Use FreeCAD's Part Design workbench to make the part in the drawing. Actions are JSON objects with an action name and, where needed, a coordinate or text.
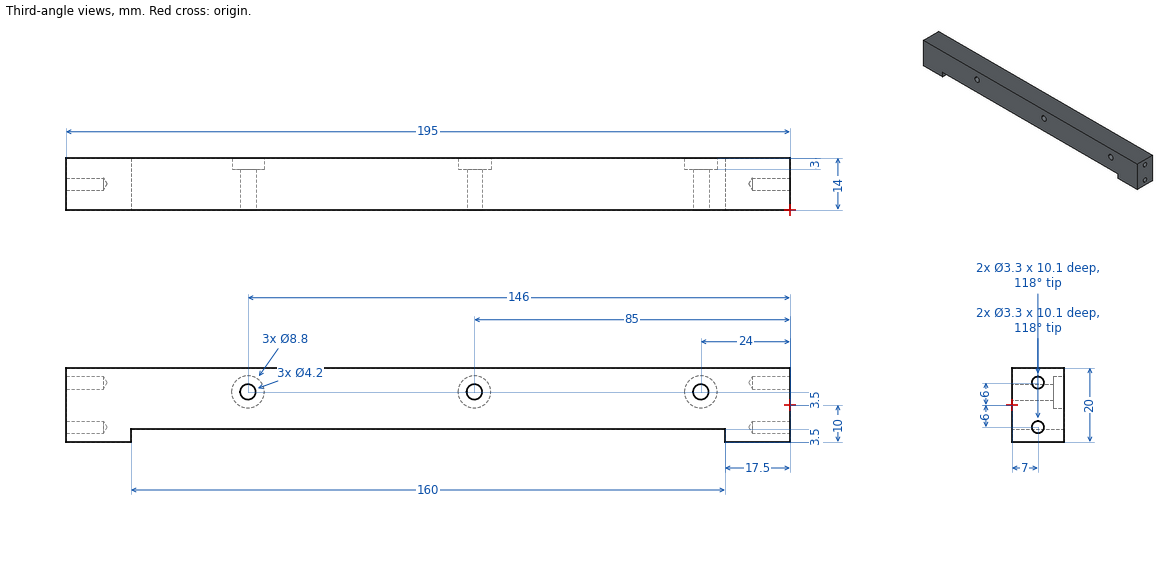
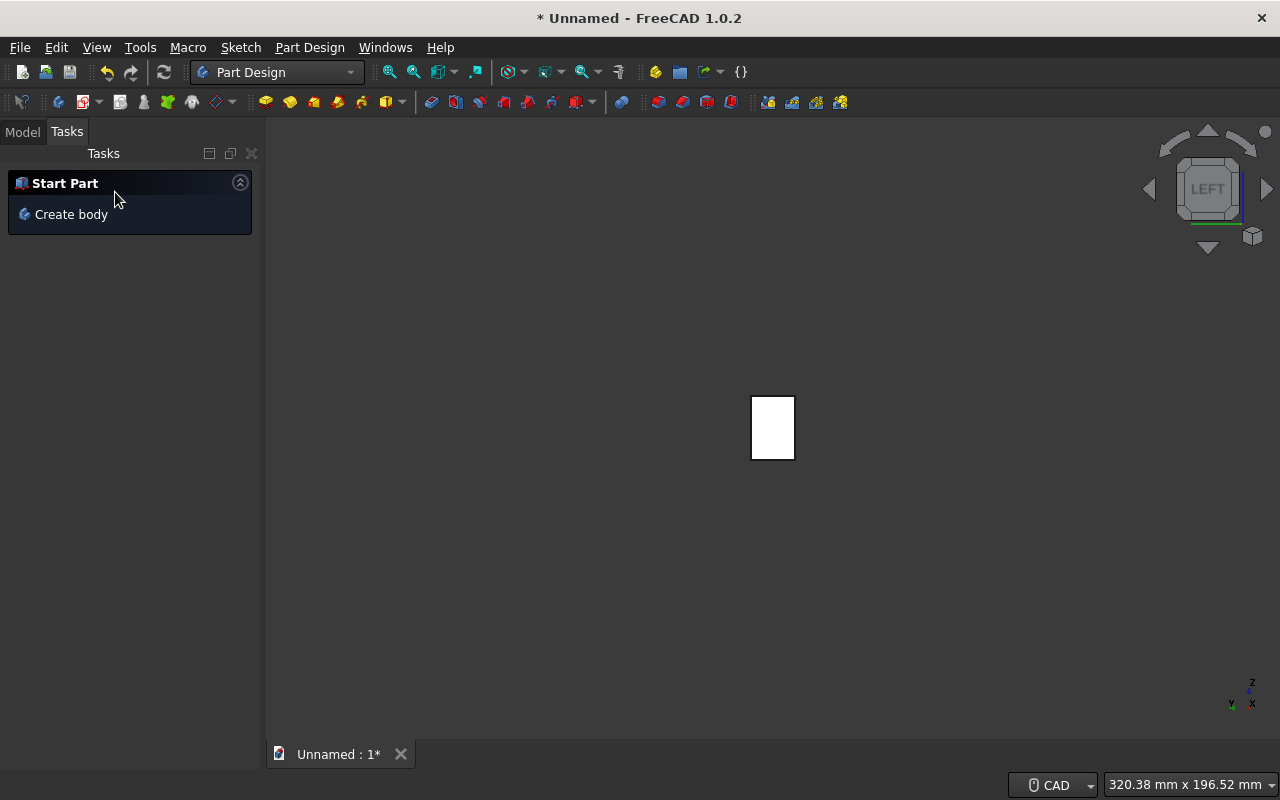
{"action": "key", "text": "v f"}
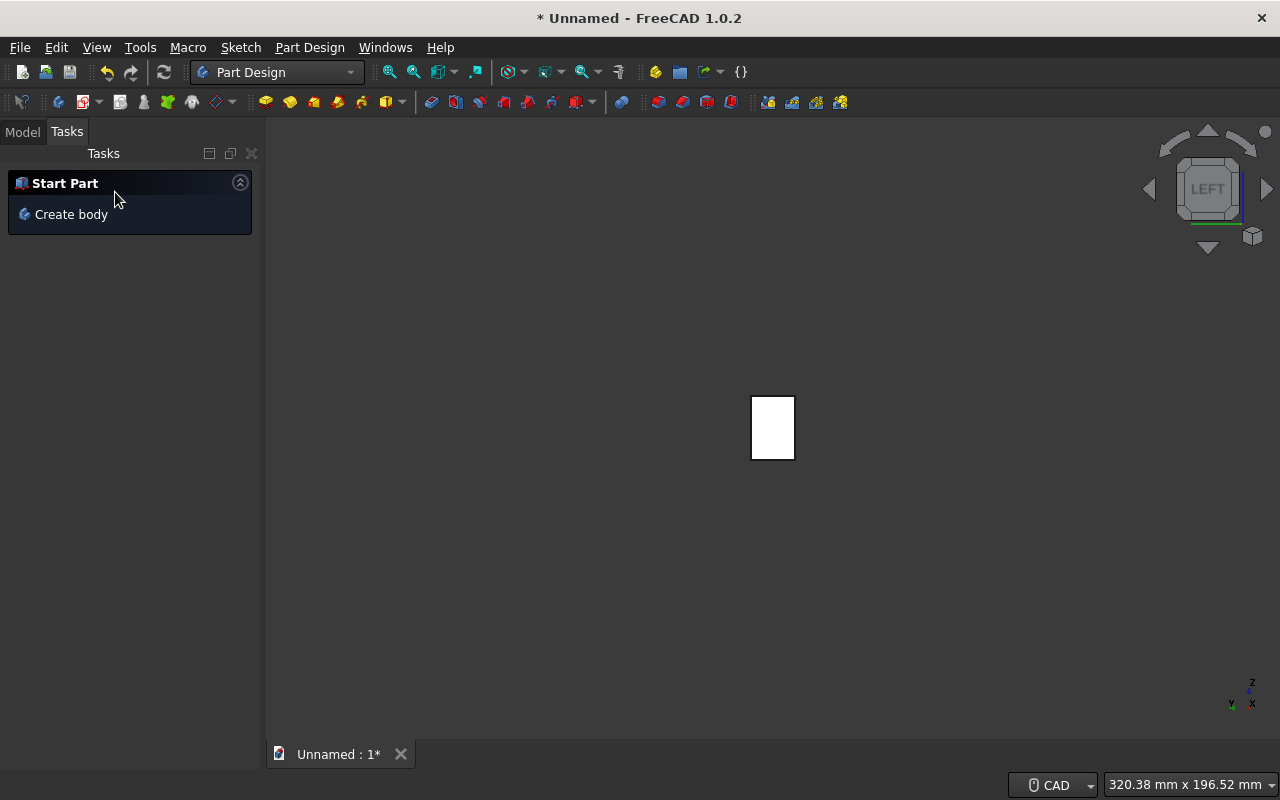
{"action": "left_click", "coordinate": [773, 418]}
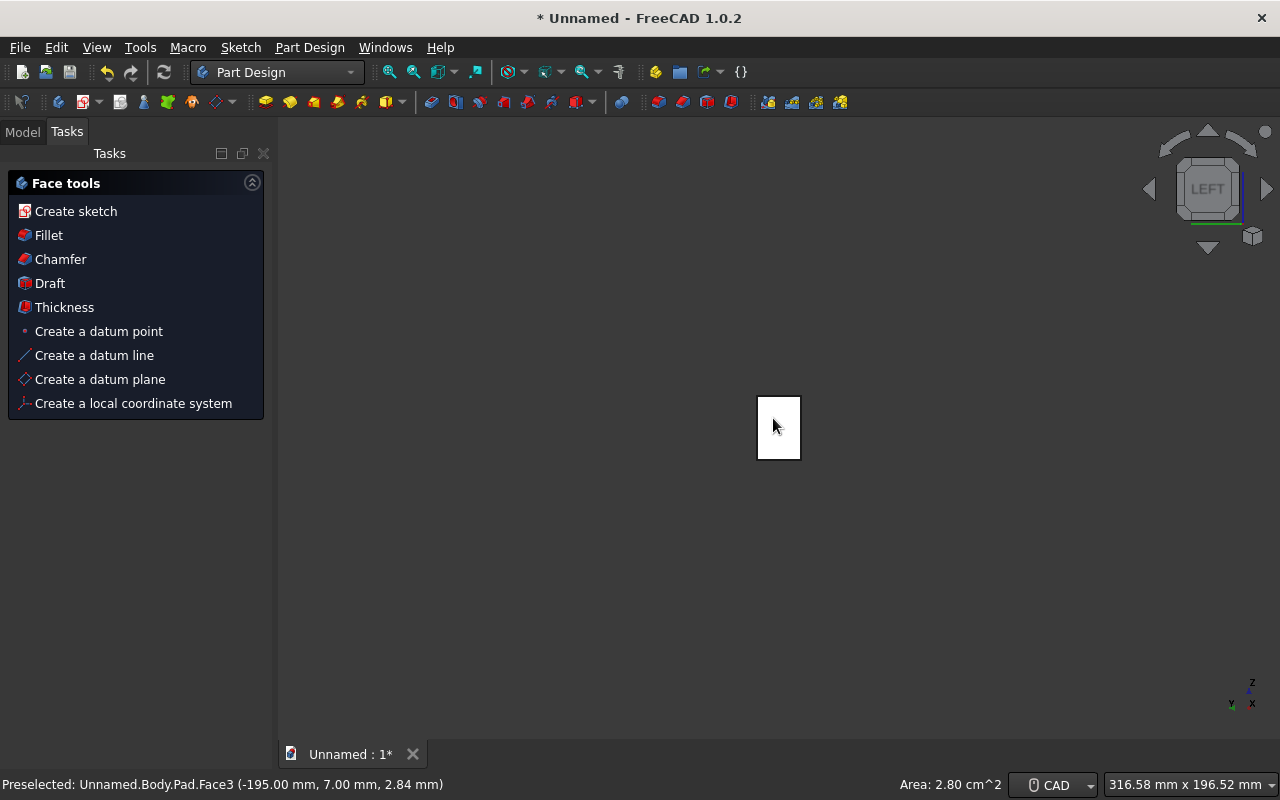
{"action": "left_click", "coordinate": [84, 102]}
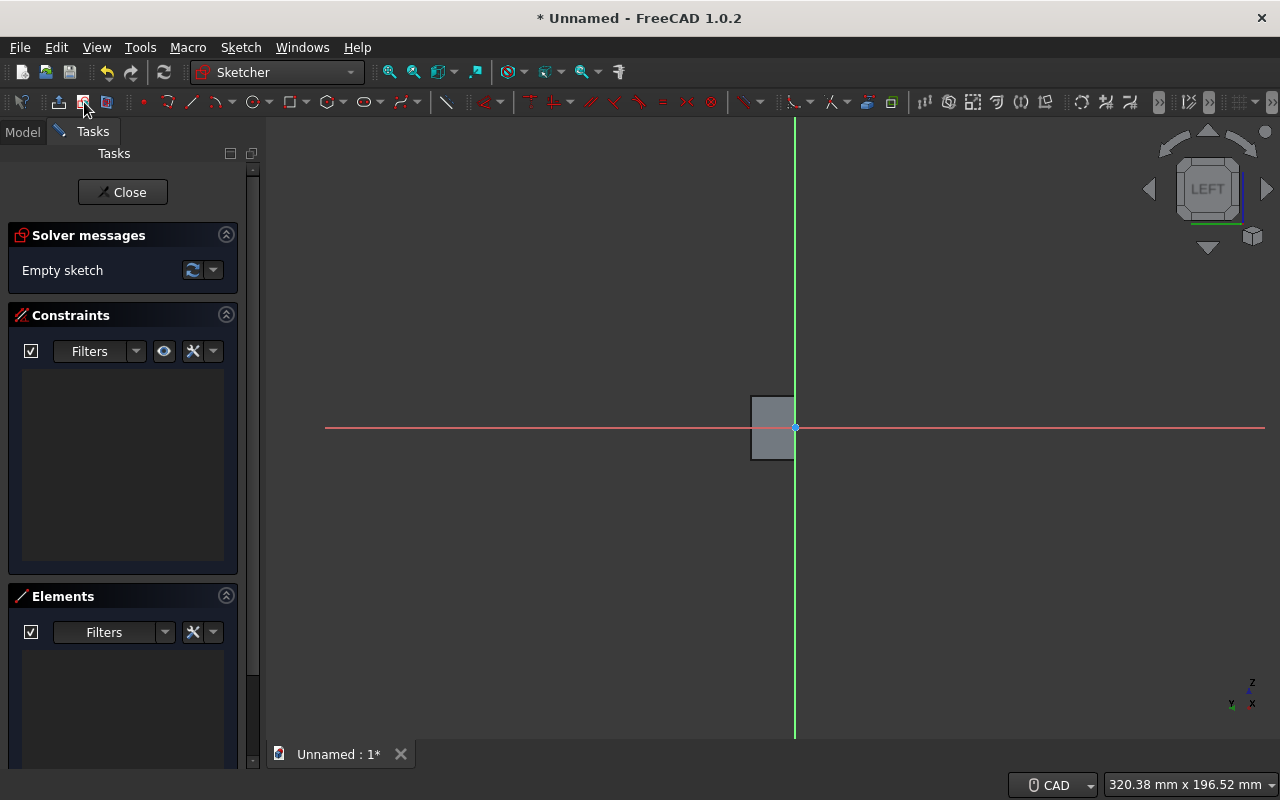
{"action": "scroll", "coordinate": [791, 428], "scroll_direction": "up", "scroll_amount": 11}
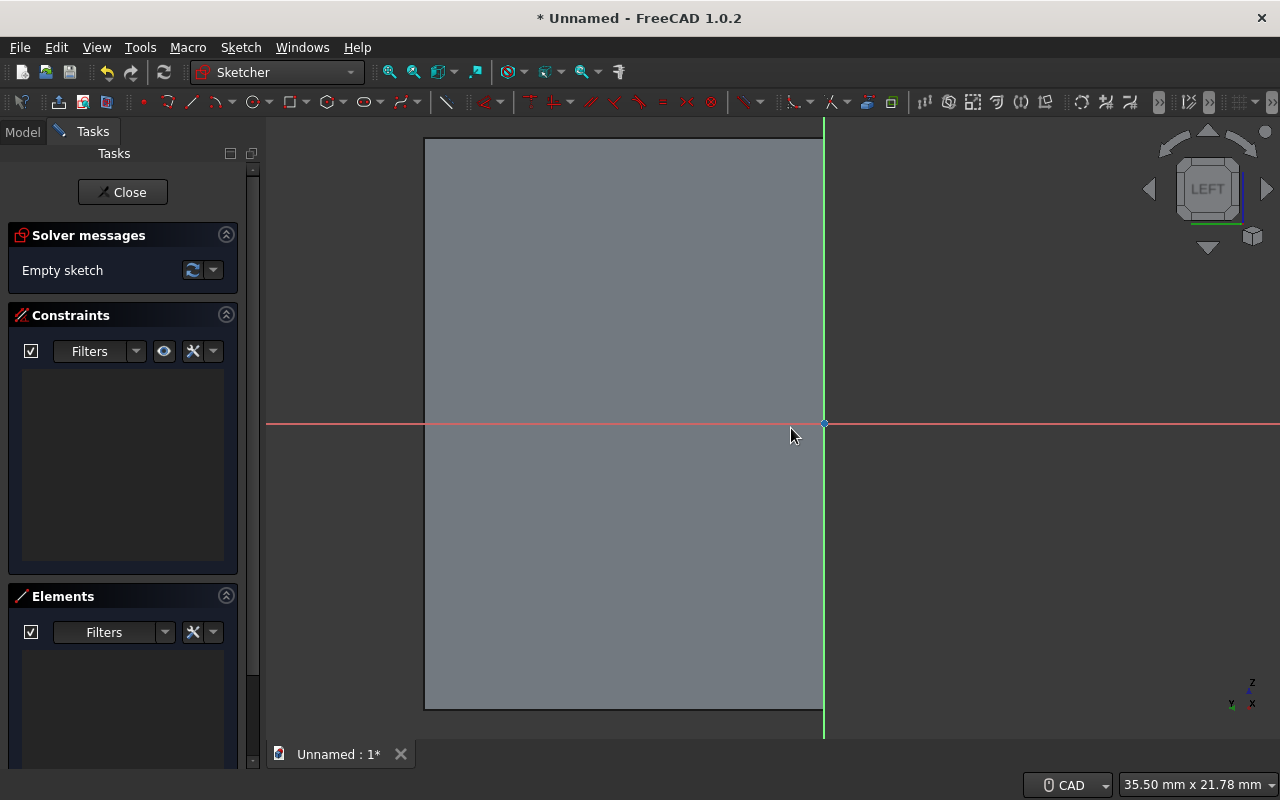
{"action": "left_click", "coordinate": [254, 102]}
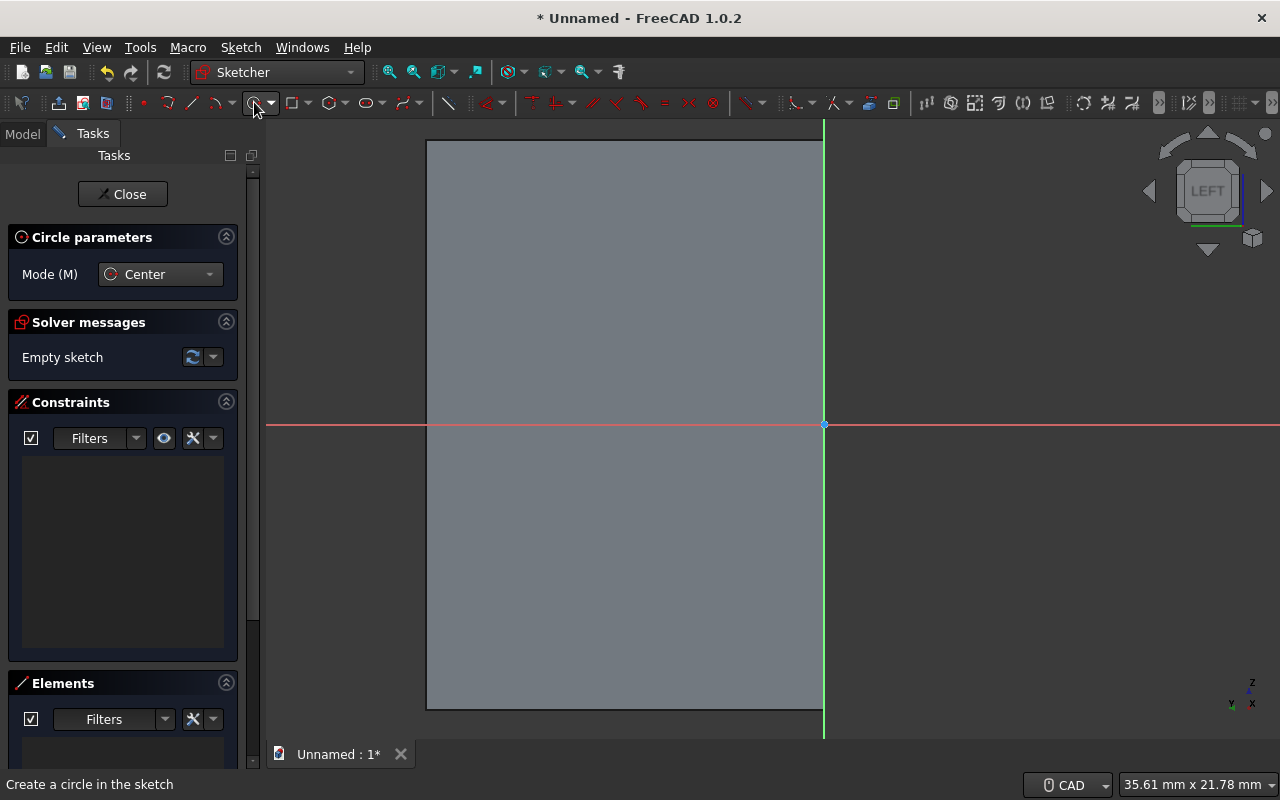
{"action": "left_click", "coordinate": [625, 596]}
{"action": "left_click", "coordinate": [658, 563]}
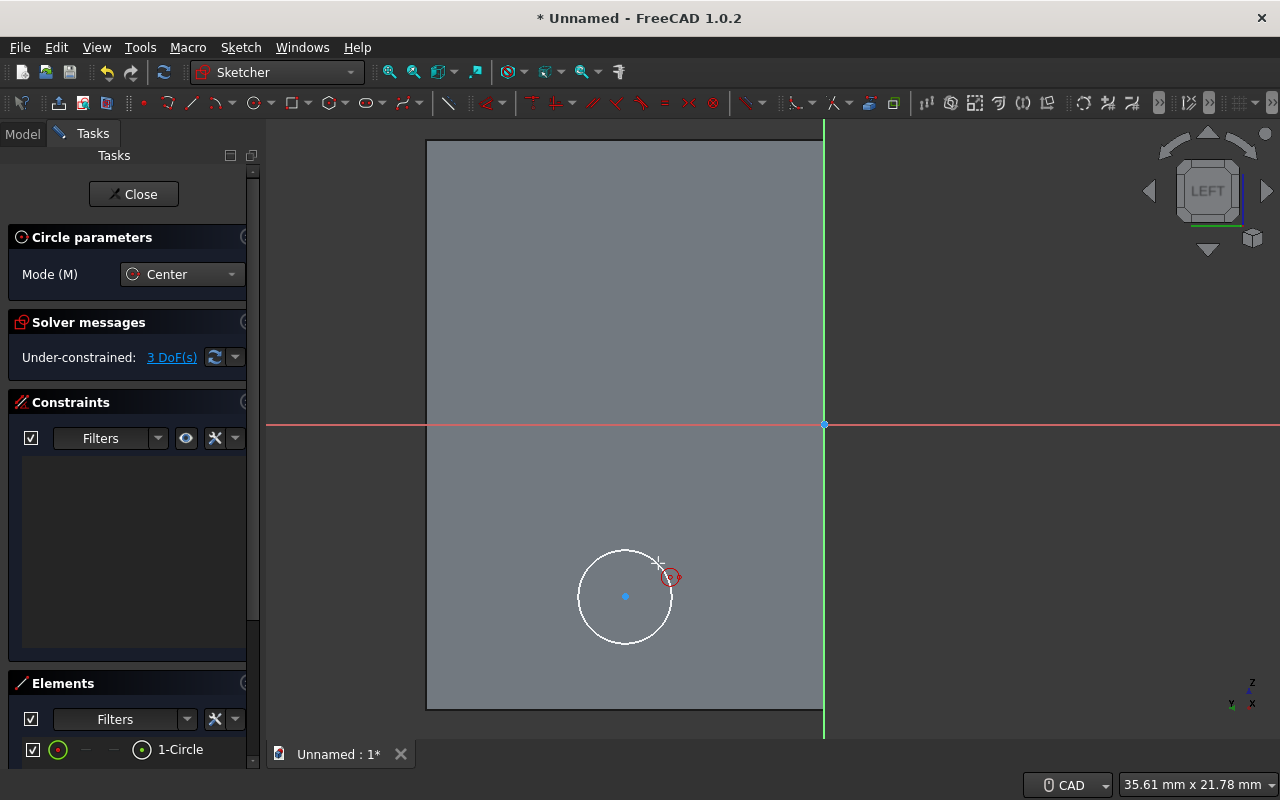
{"action": "left_click", "coordinate": [625, 254]}
{"action": "left_click", "coordinate": [658, 221]}
{"action": "key", "text": "Escape"}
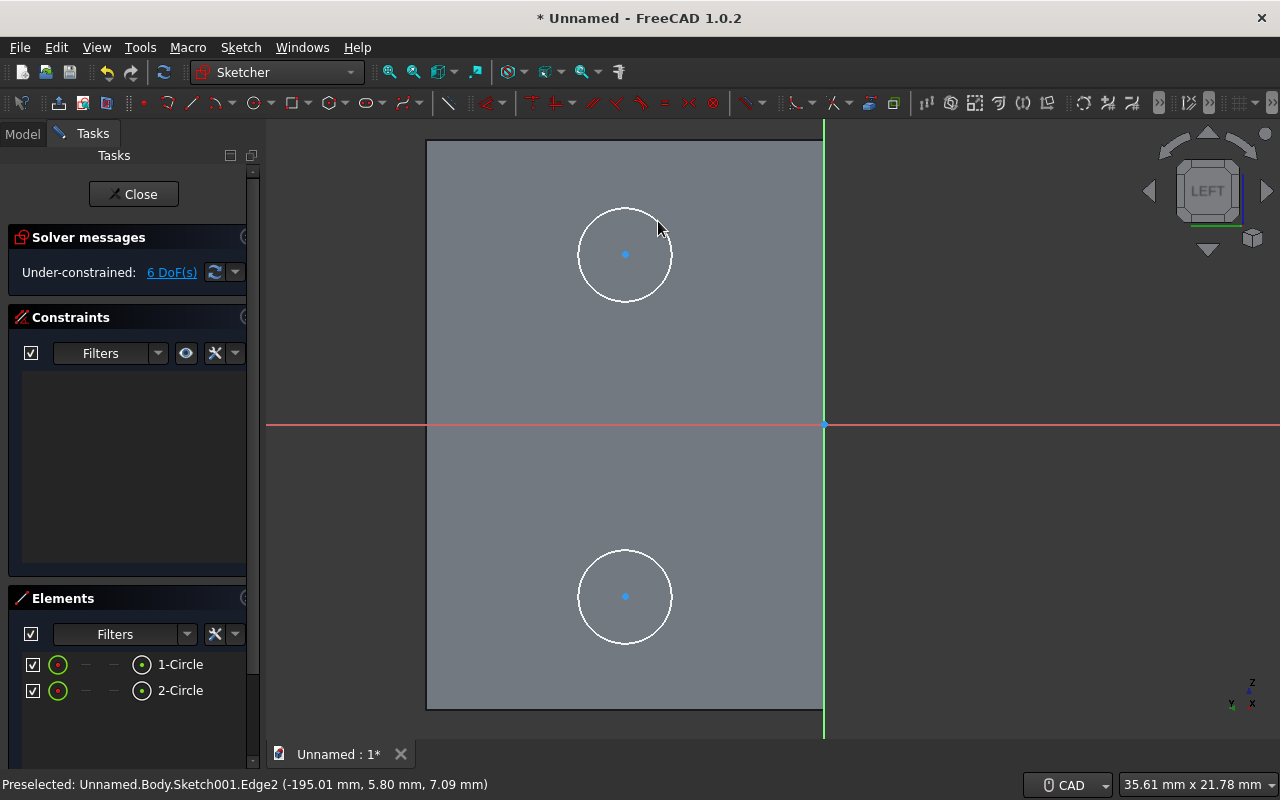
{"action": "left_click", "coordinate": [658, 564]}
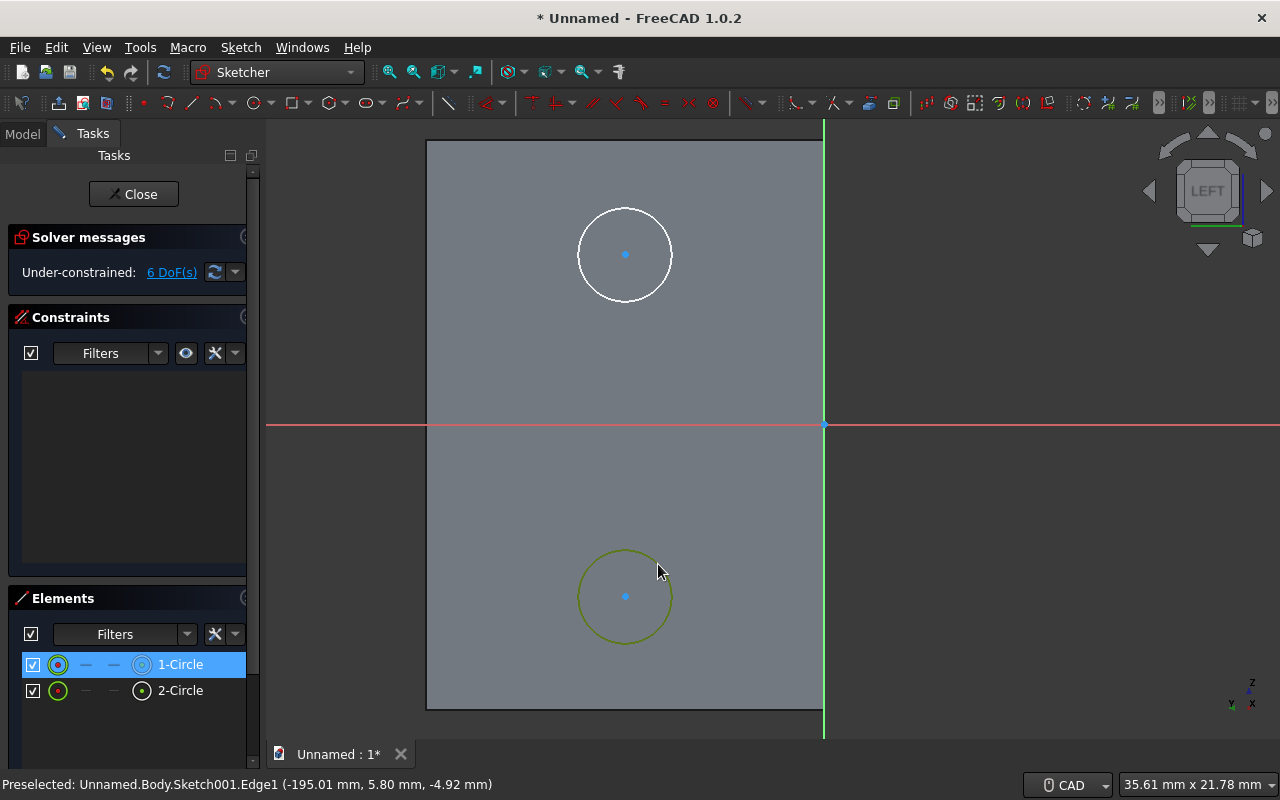
{"action": "left_click", "coordinate": [658, 222]}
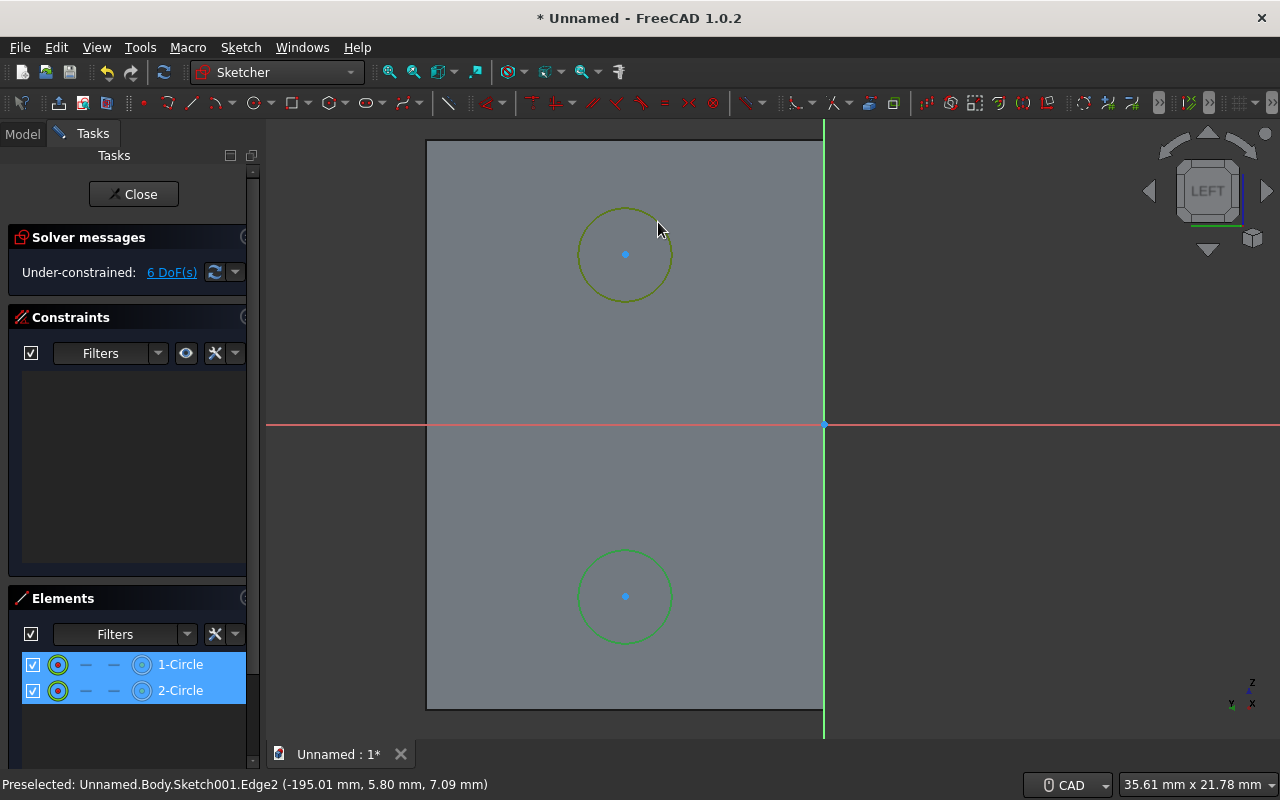
{"action": "key", "text": "e"}